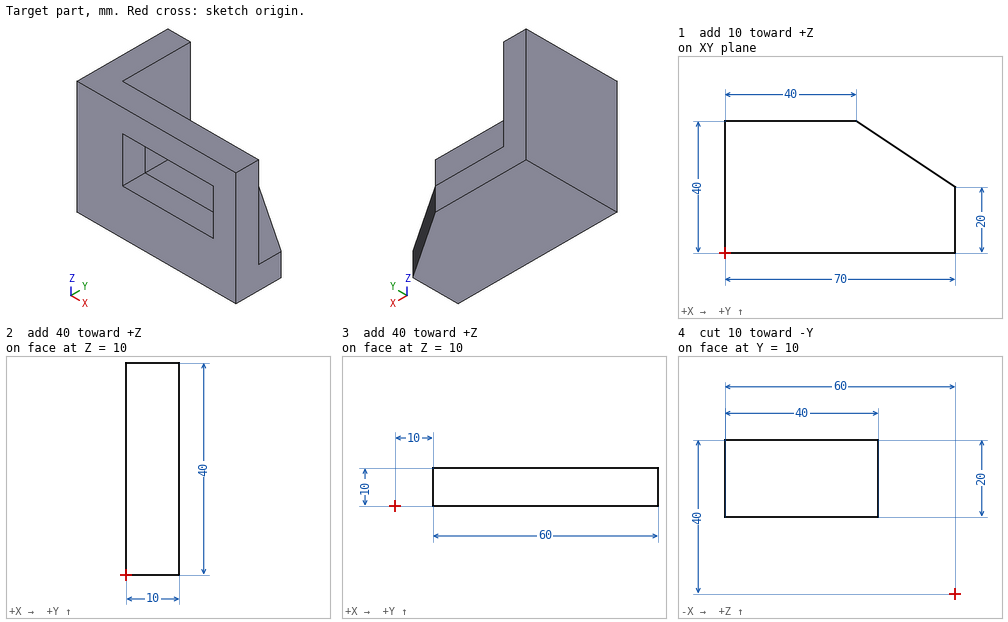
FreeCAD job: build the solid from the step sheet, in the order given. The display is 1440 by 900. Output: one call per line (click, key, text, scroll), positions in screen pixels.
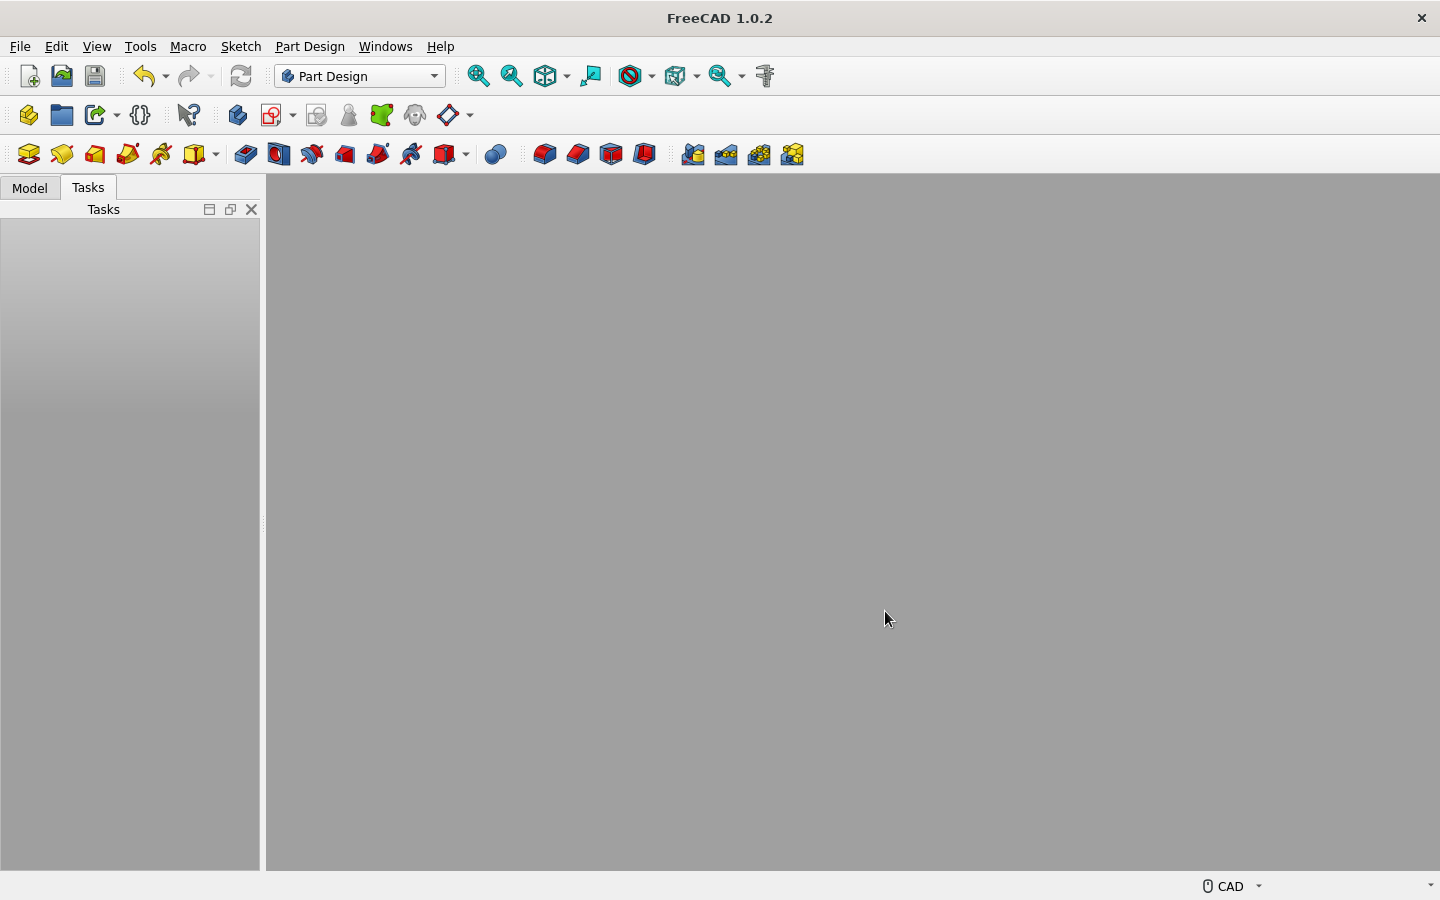
click(29, 76)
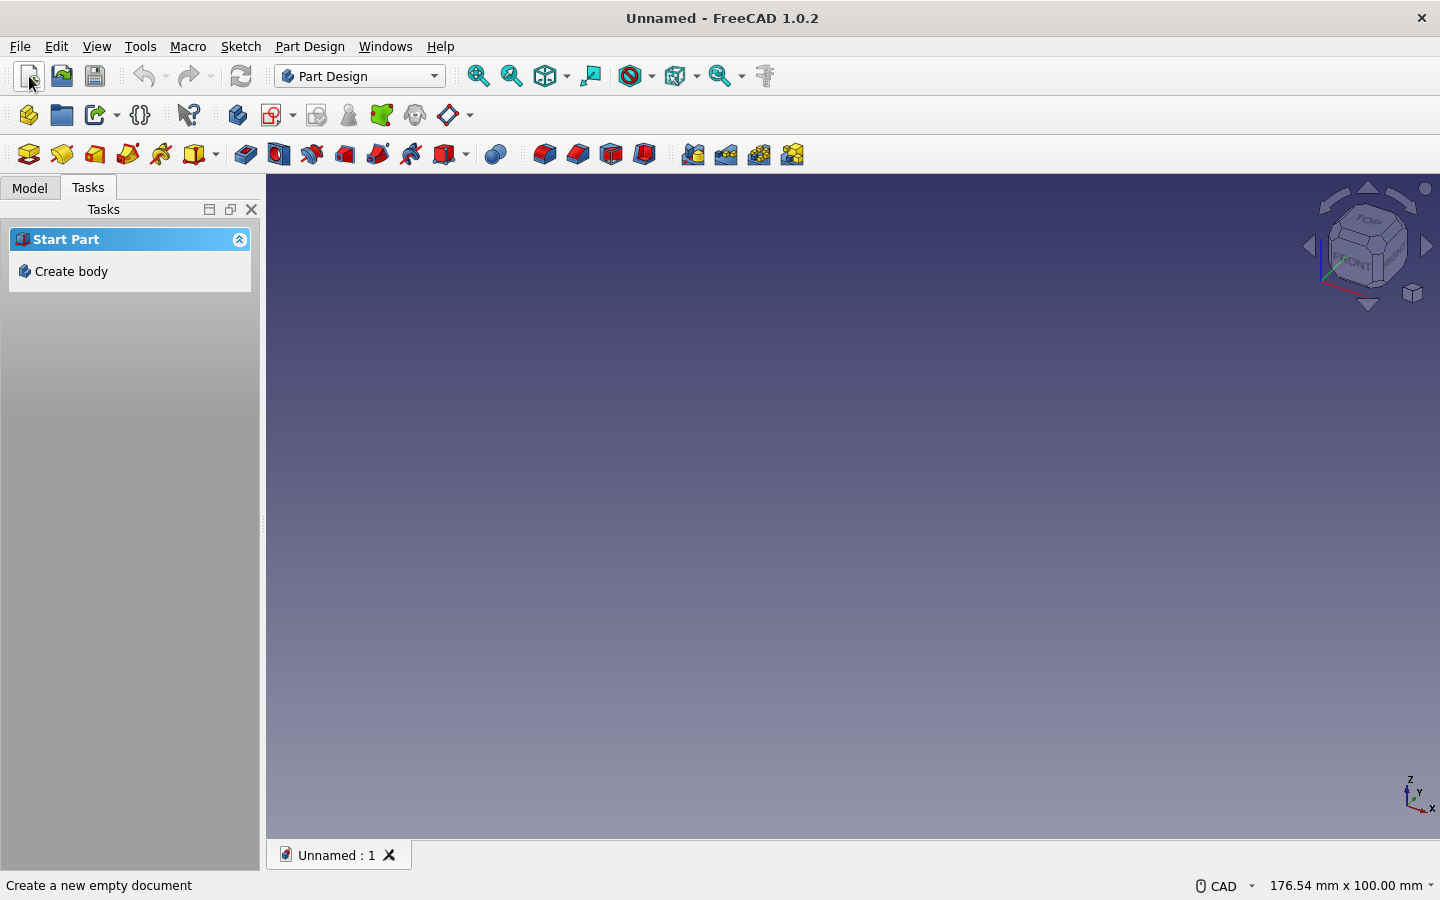
click(270, 116)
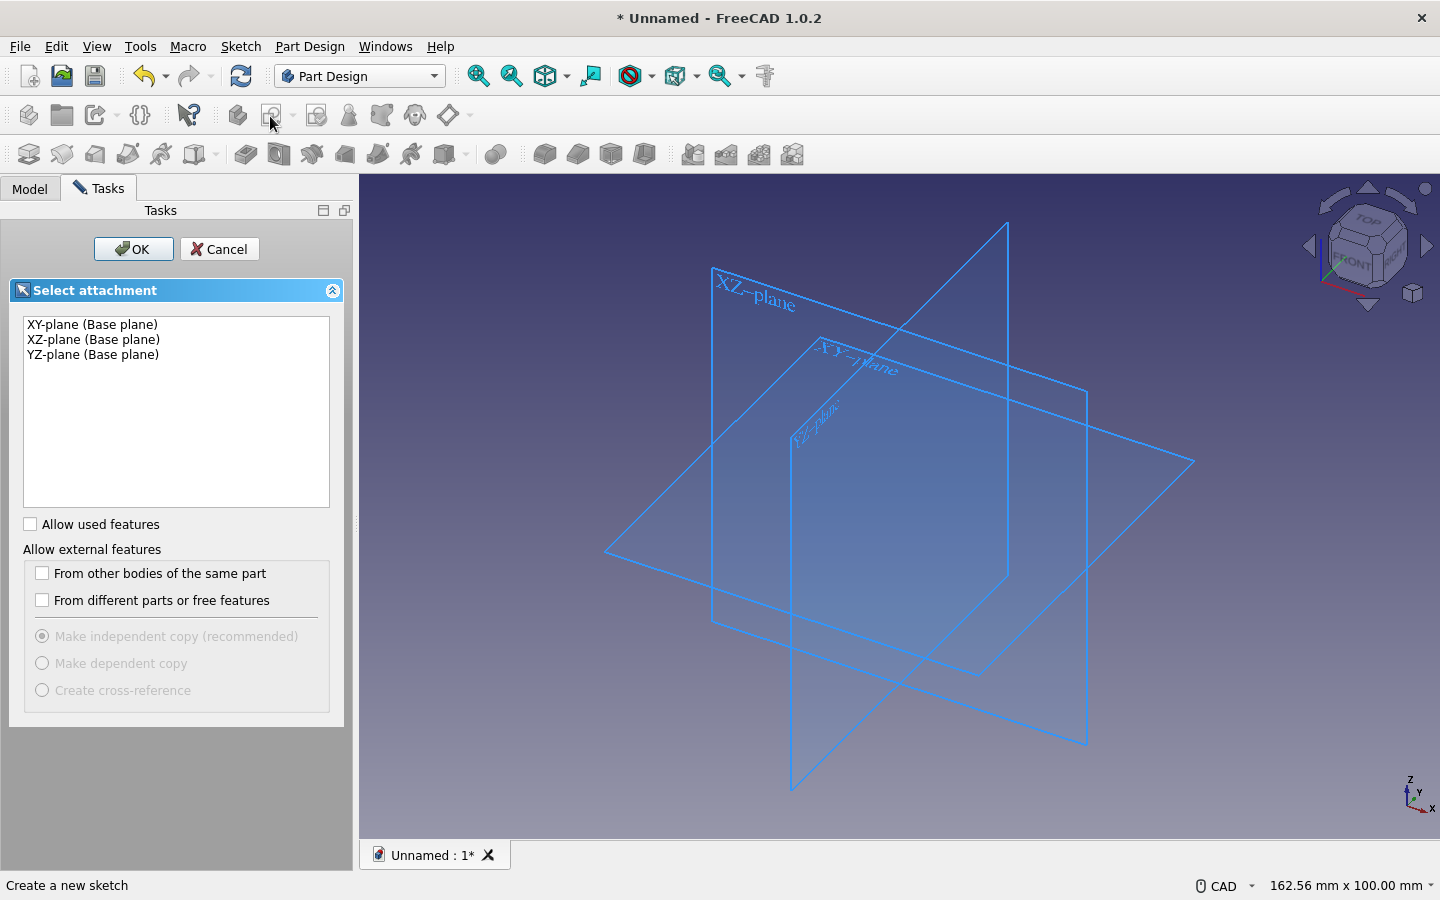
click(84, 324)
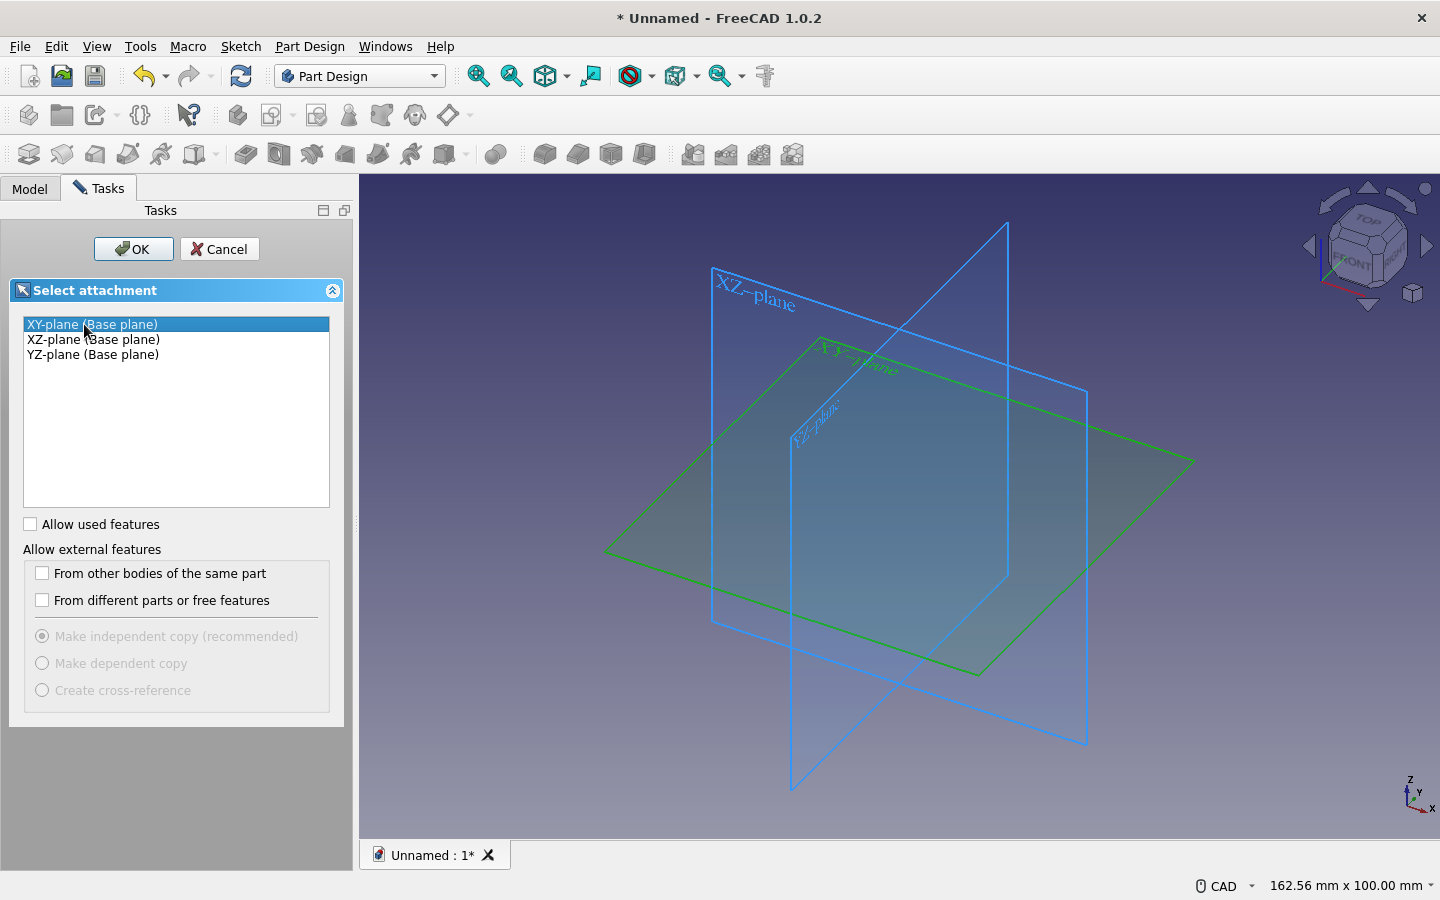
click(134, 249)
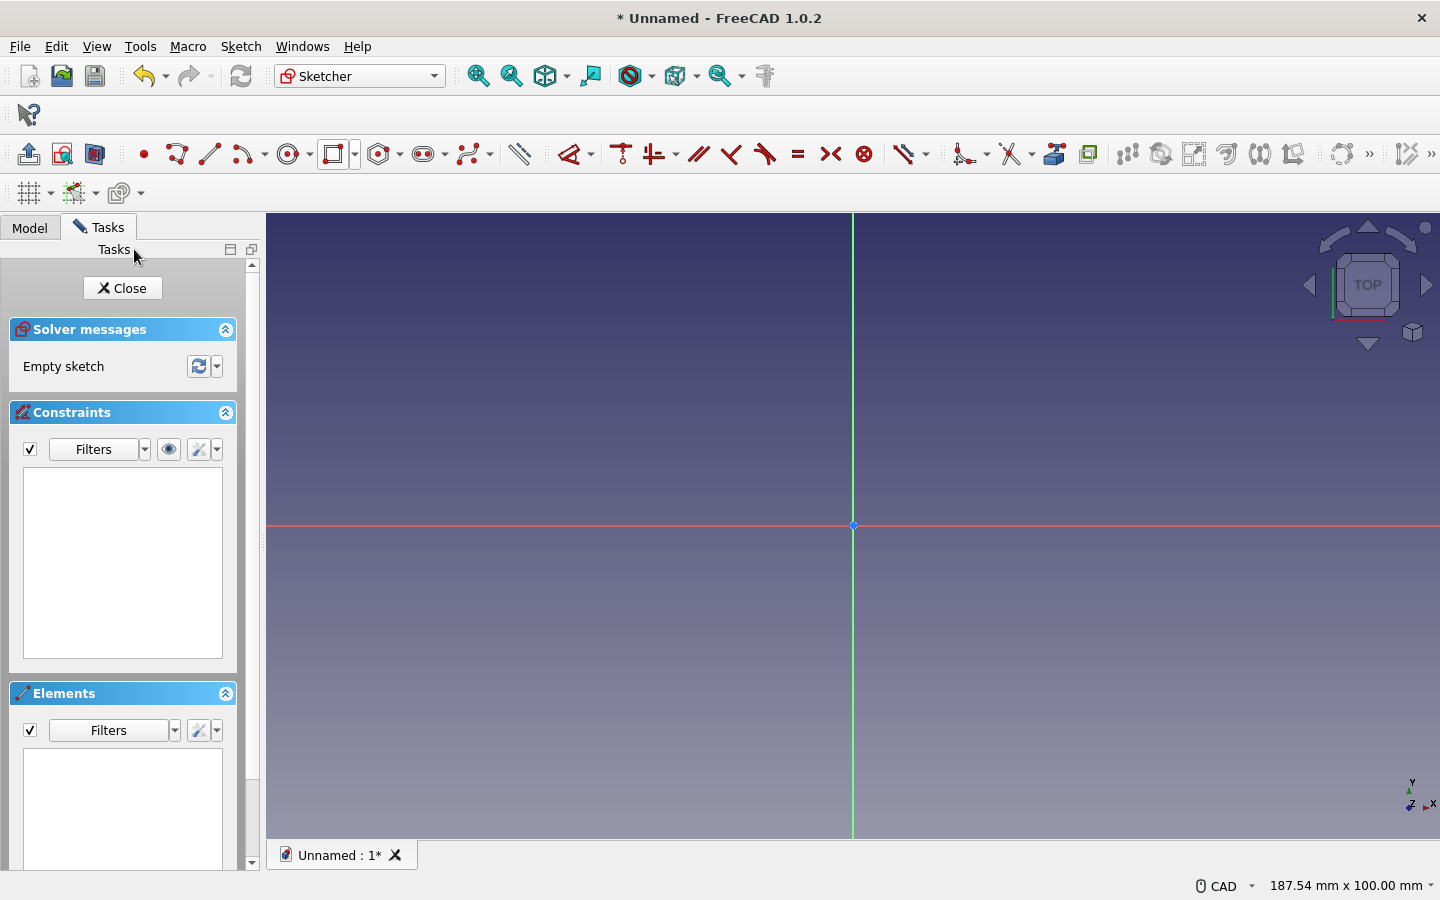
scroll(294, 811, down, 1)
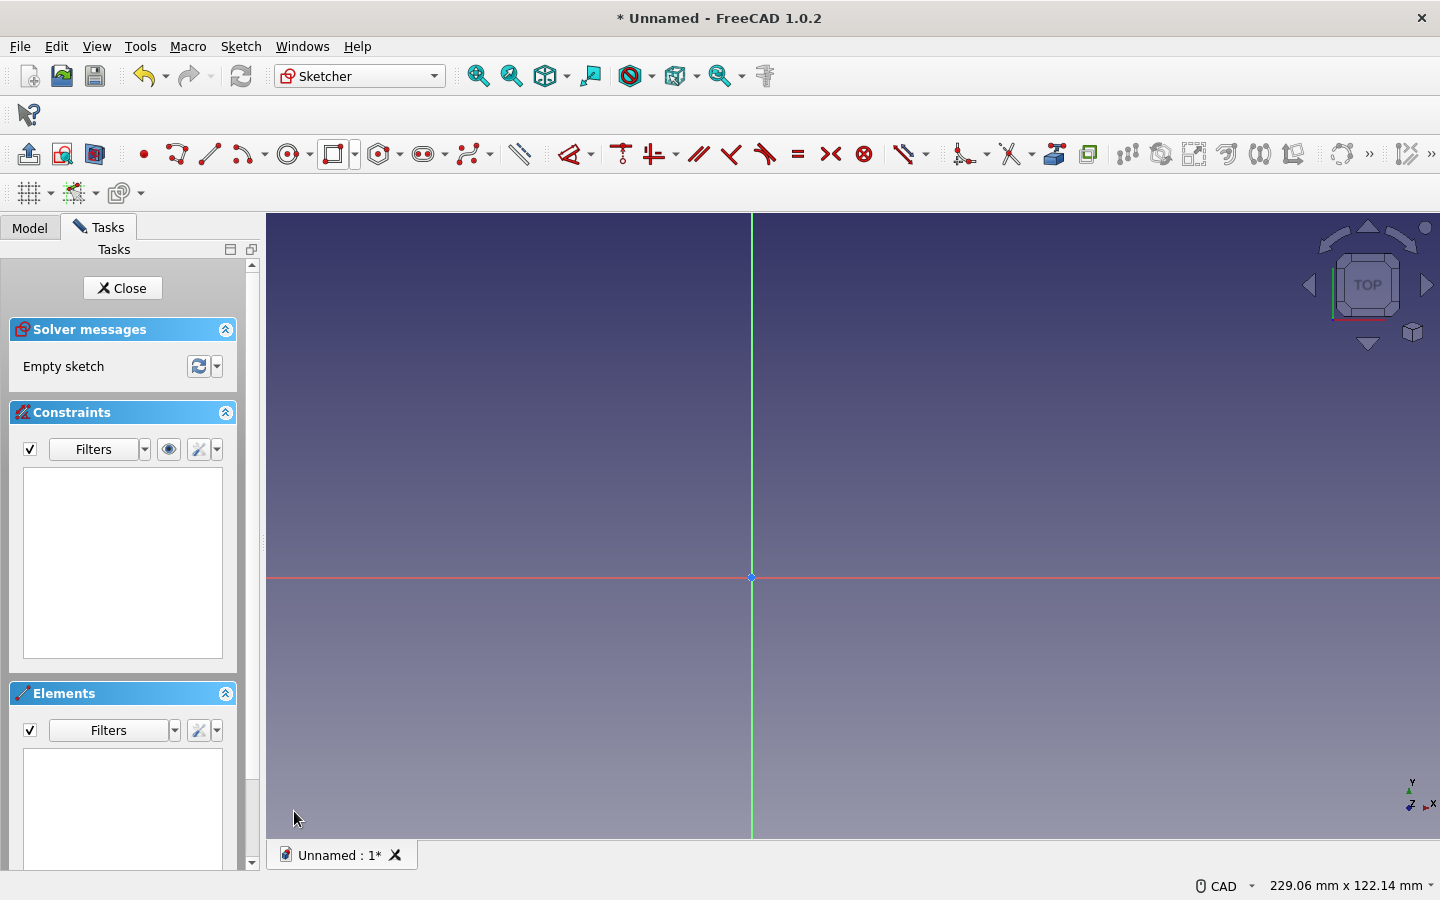
scroll(1109, 414, up, 3)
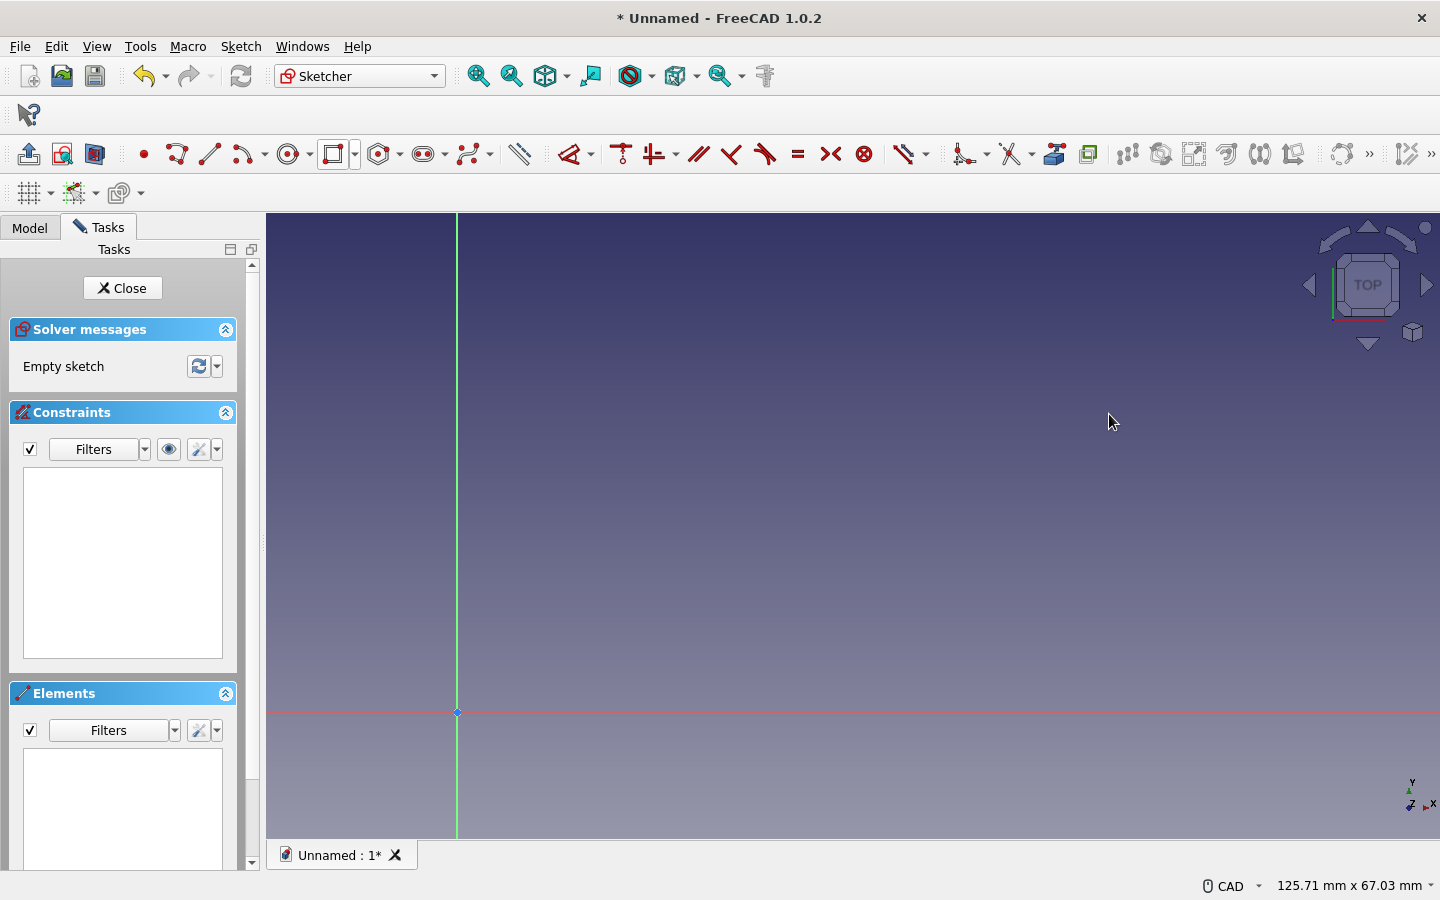
key(g)
key(m)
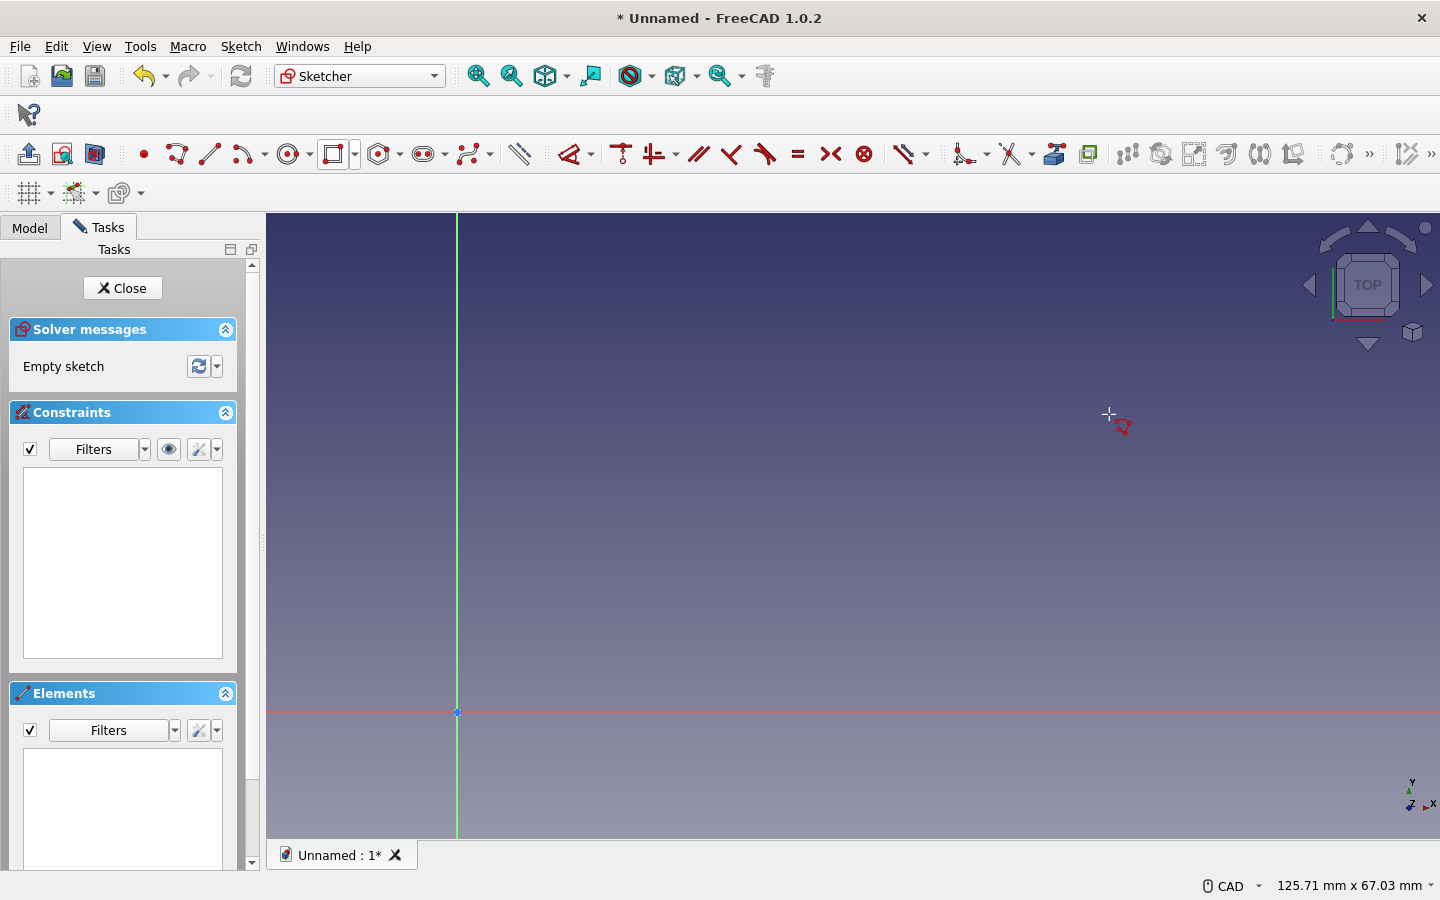
click(457, 712)
click(1111, 703)
click(1111, 525)
click(831, 339)
click(466, 339)
click(457, 712)
key(Escape)
key(Escape)